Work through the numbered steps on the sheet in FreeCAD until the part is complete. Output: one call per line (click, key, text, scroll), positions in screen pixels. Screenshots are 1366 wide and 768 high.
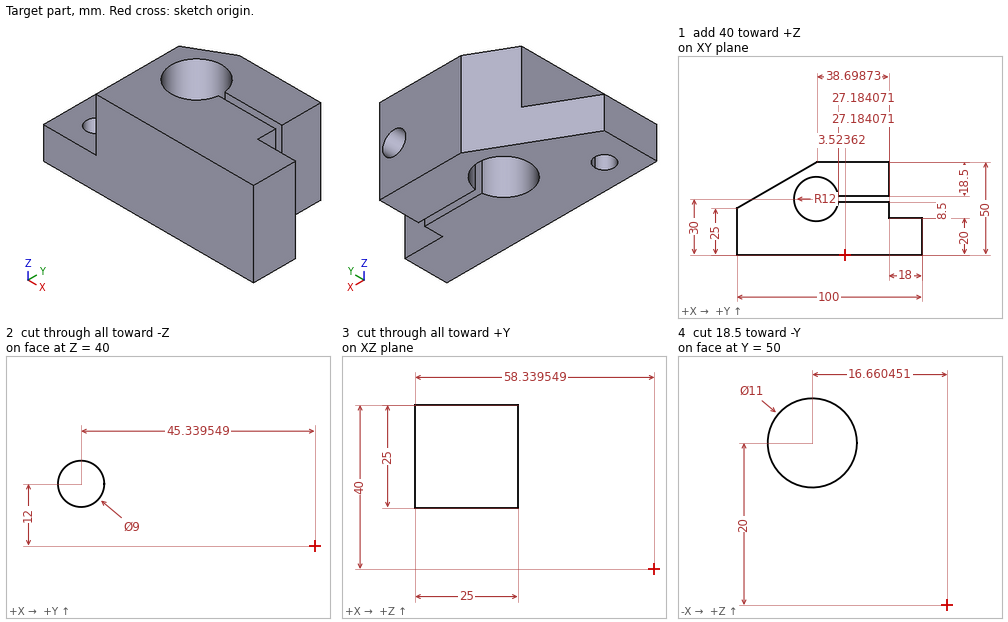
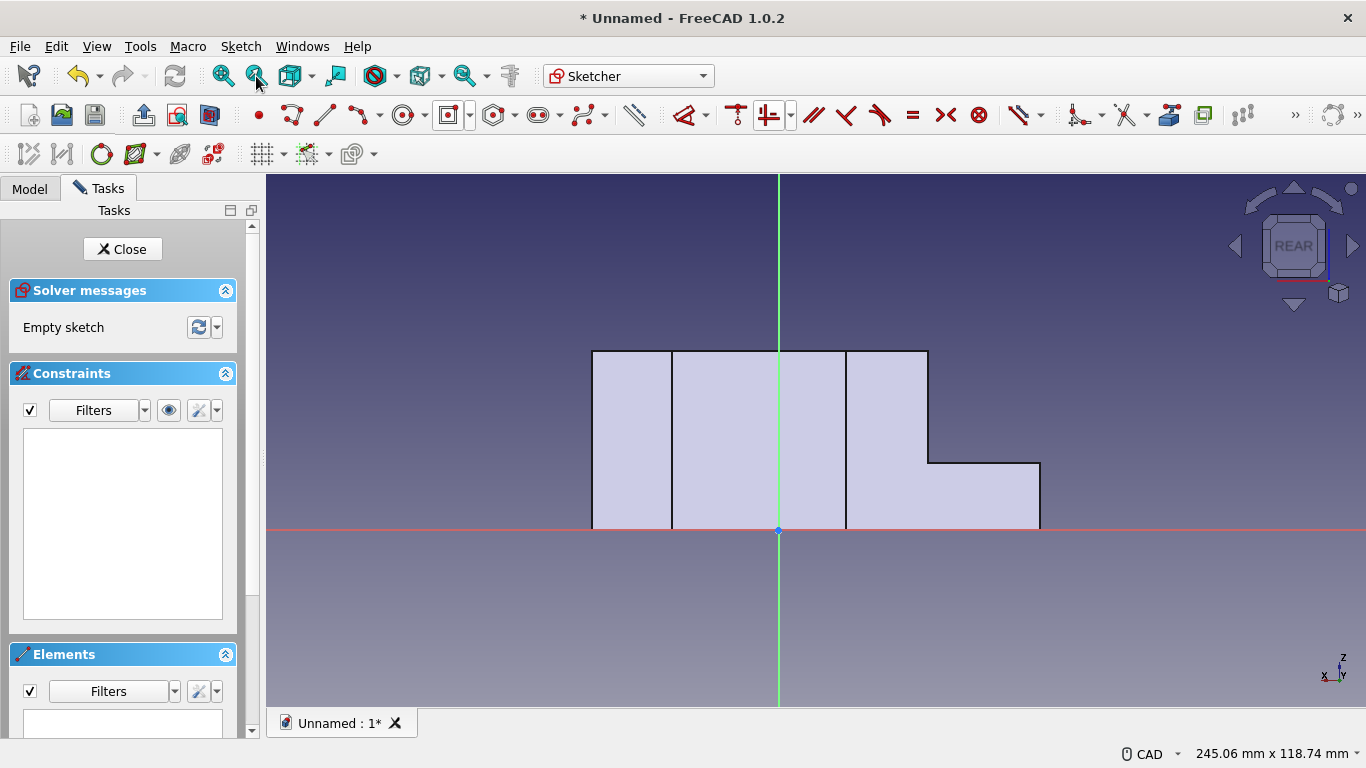
scroll(718, 492, up, 5)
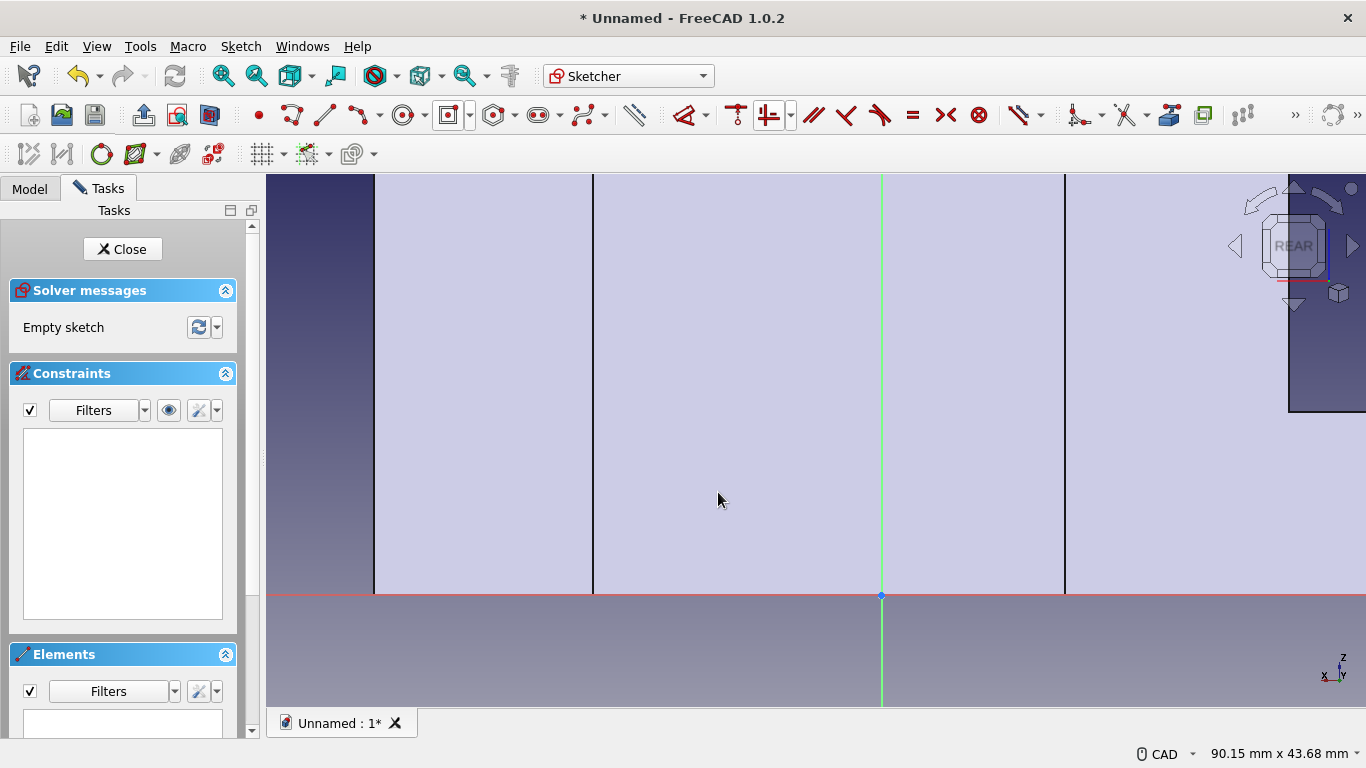
key(g)
key(c)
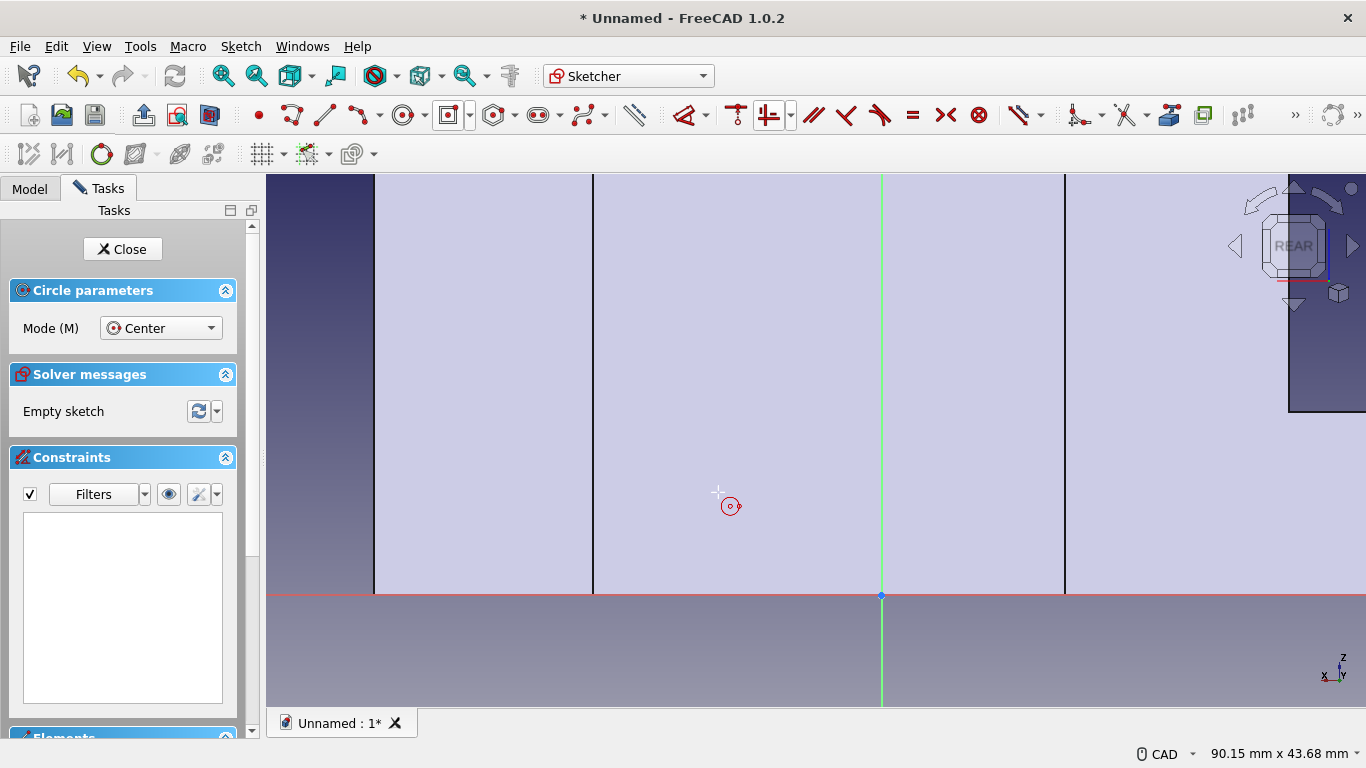
click(679, 351)
move(726, 304)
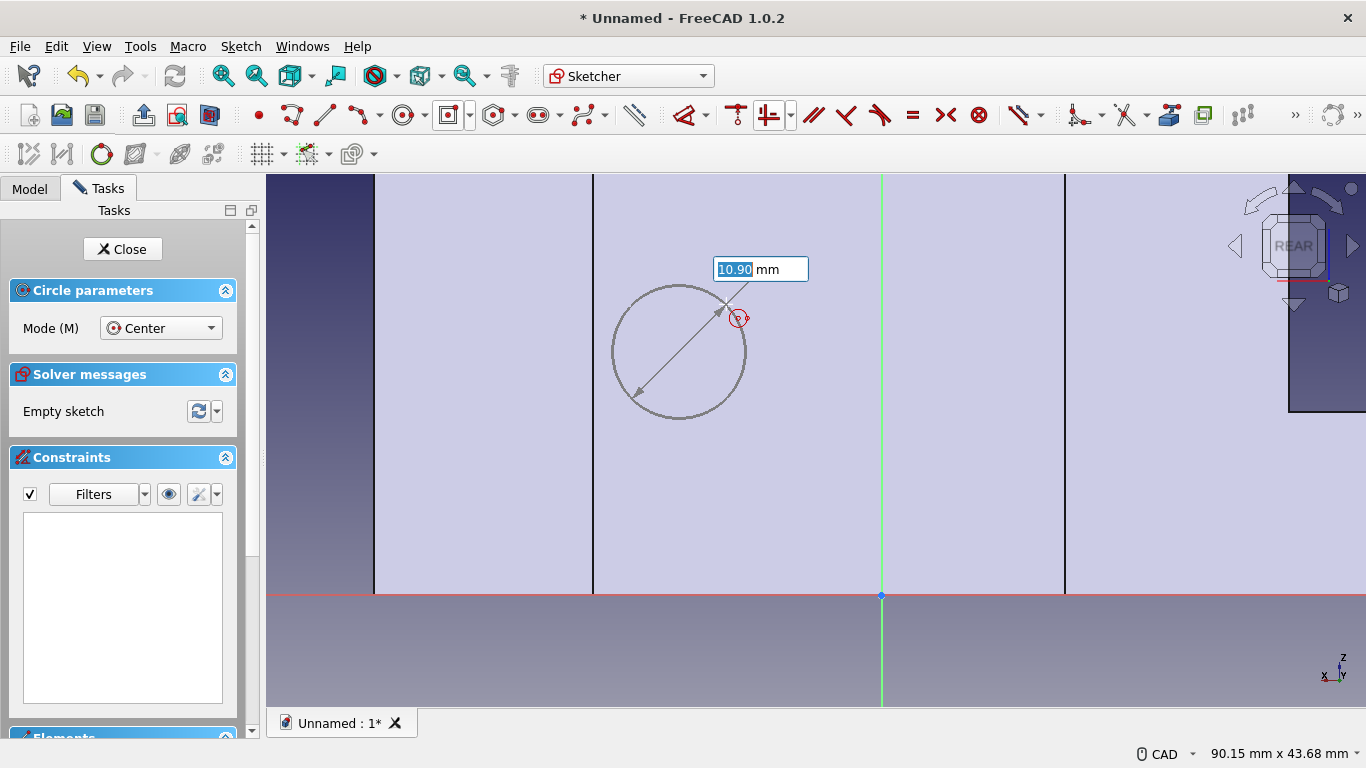
text(11)
key(Return)
key(Escape)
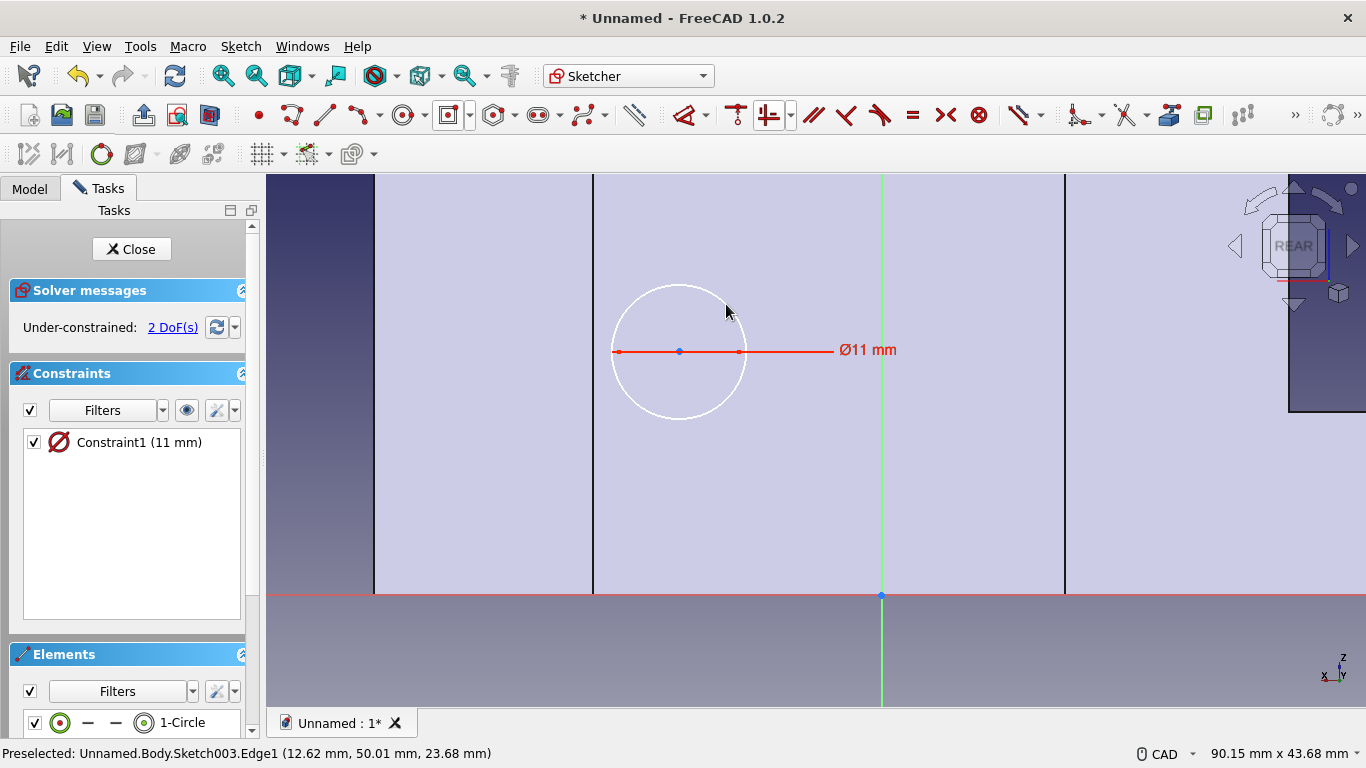
click(684, 116)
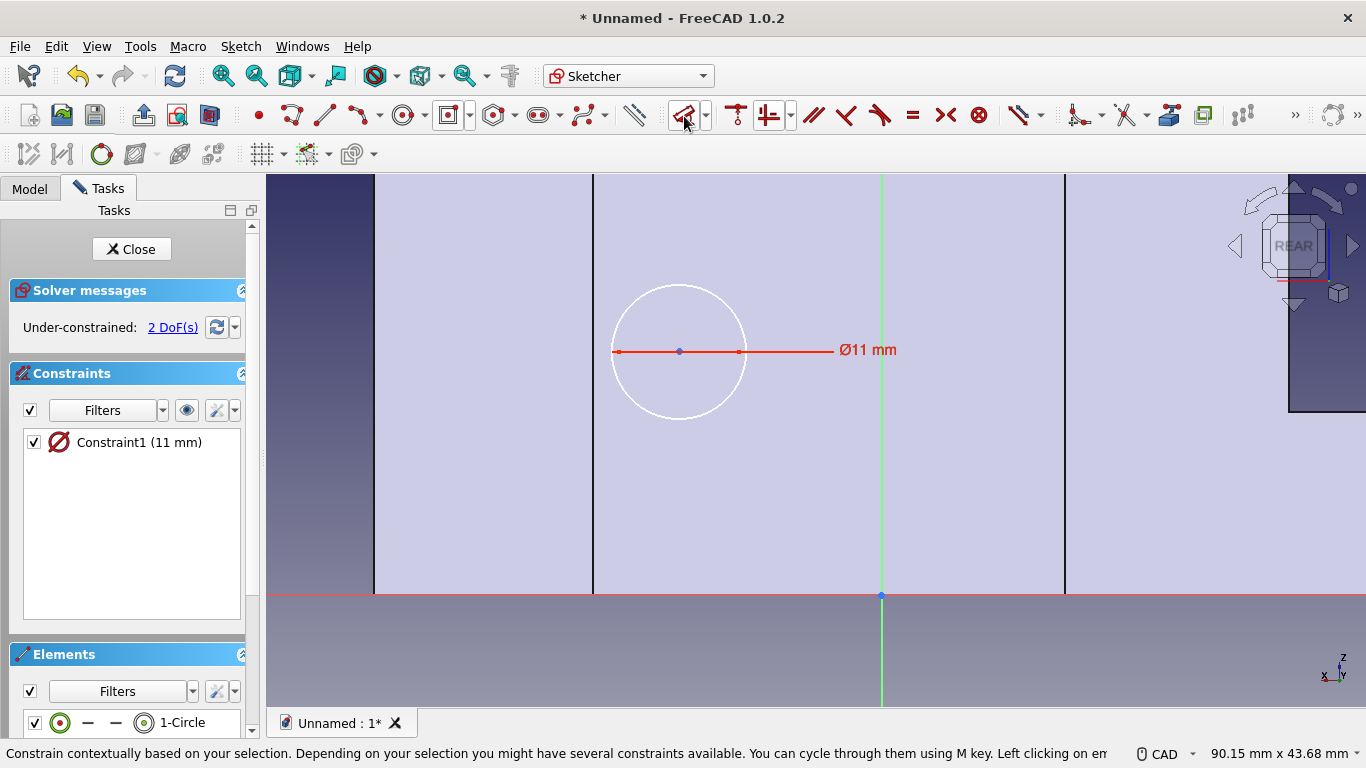
click(679, 352)
click(916, 474)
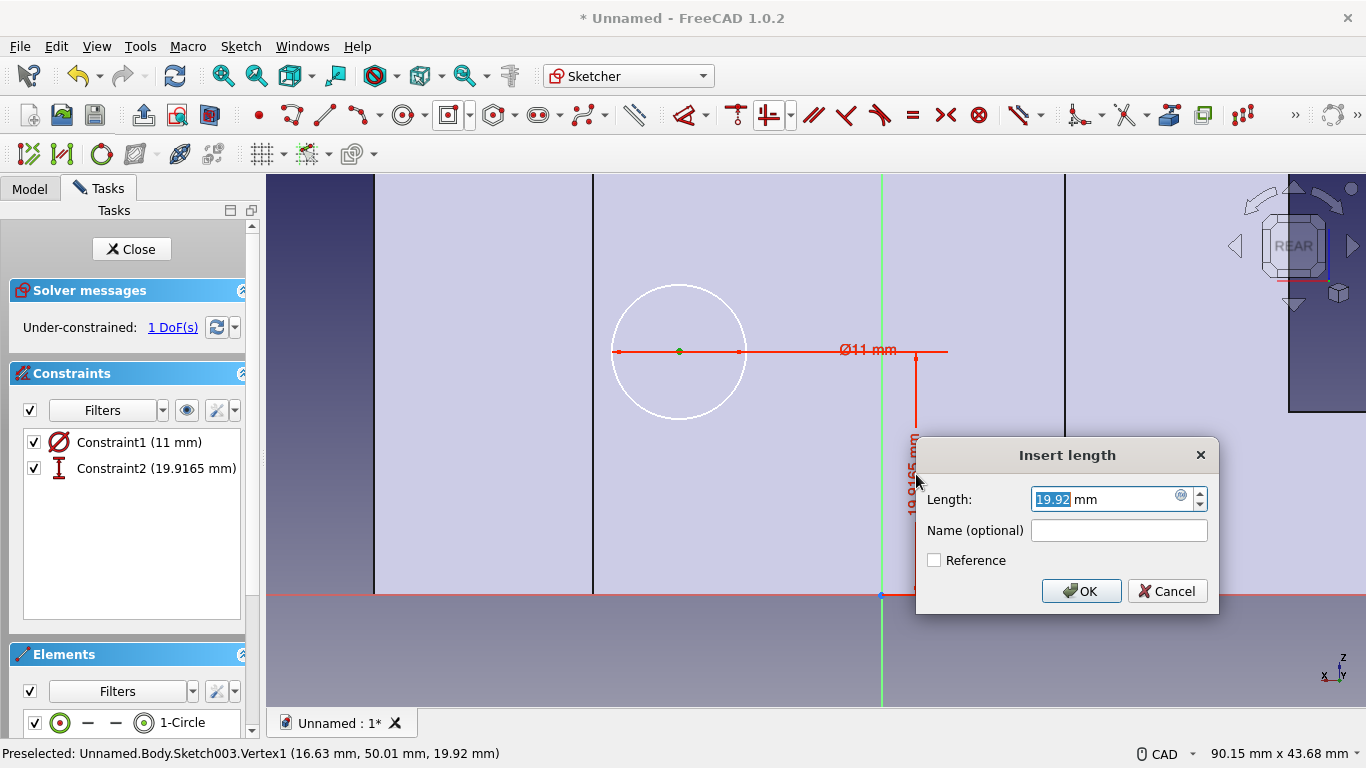
text(20)
key(Return)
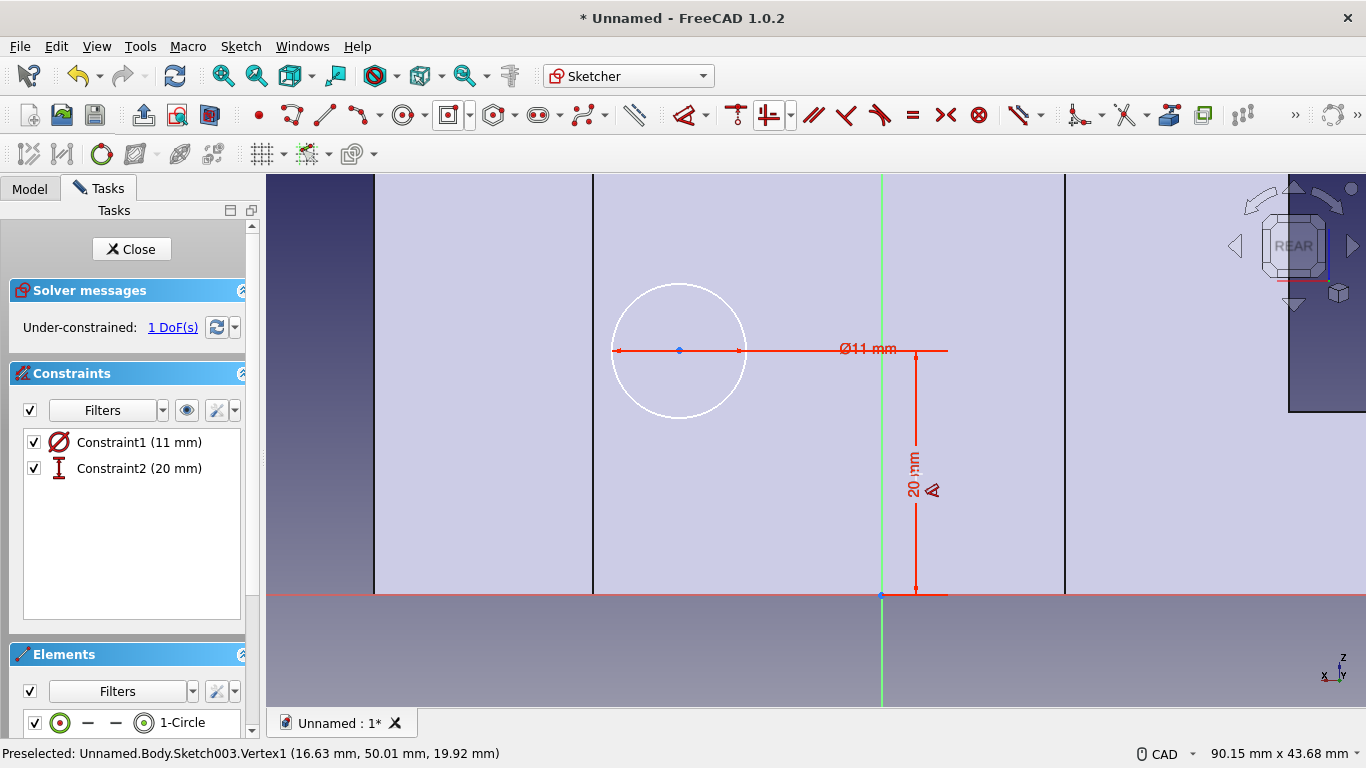
click(679, 351)
click(780, 629)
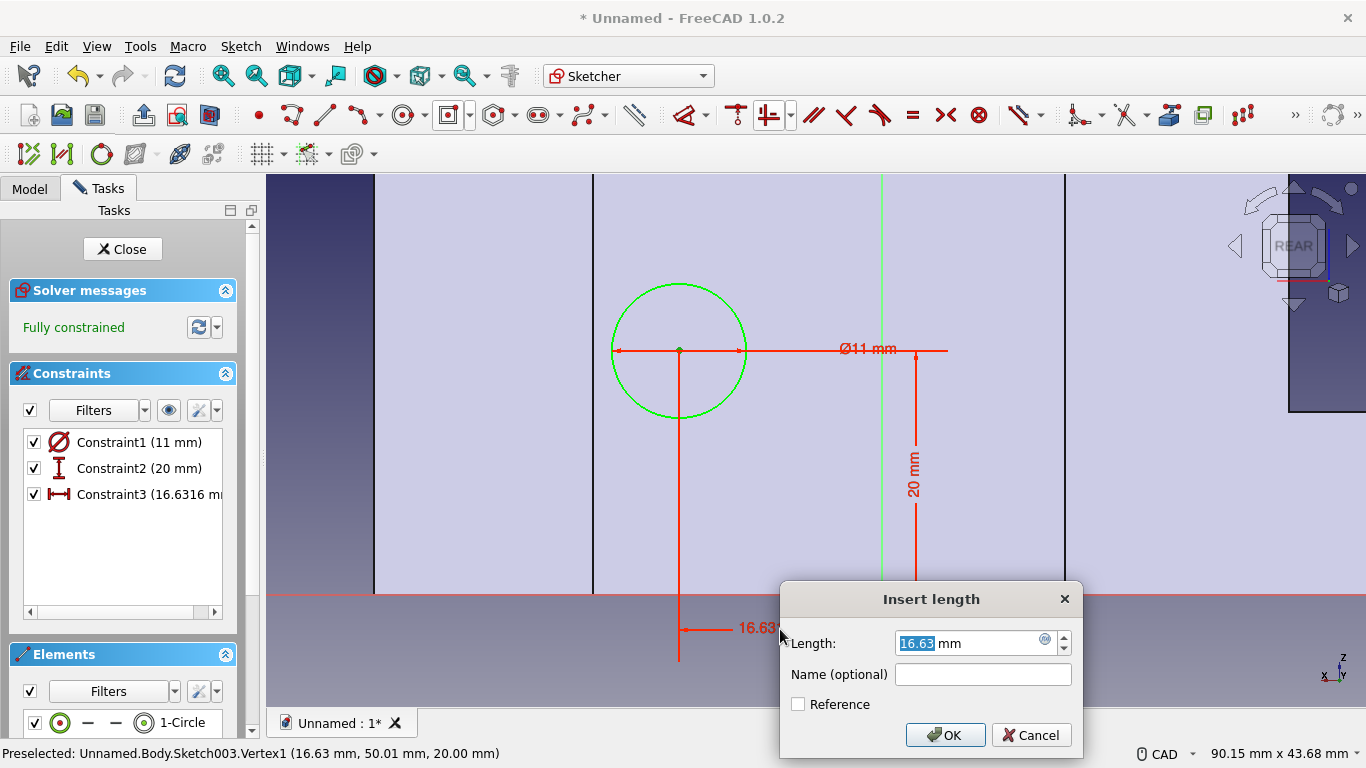
text(16.660451)
key(Return)
key(Escape)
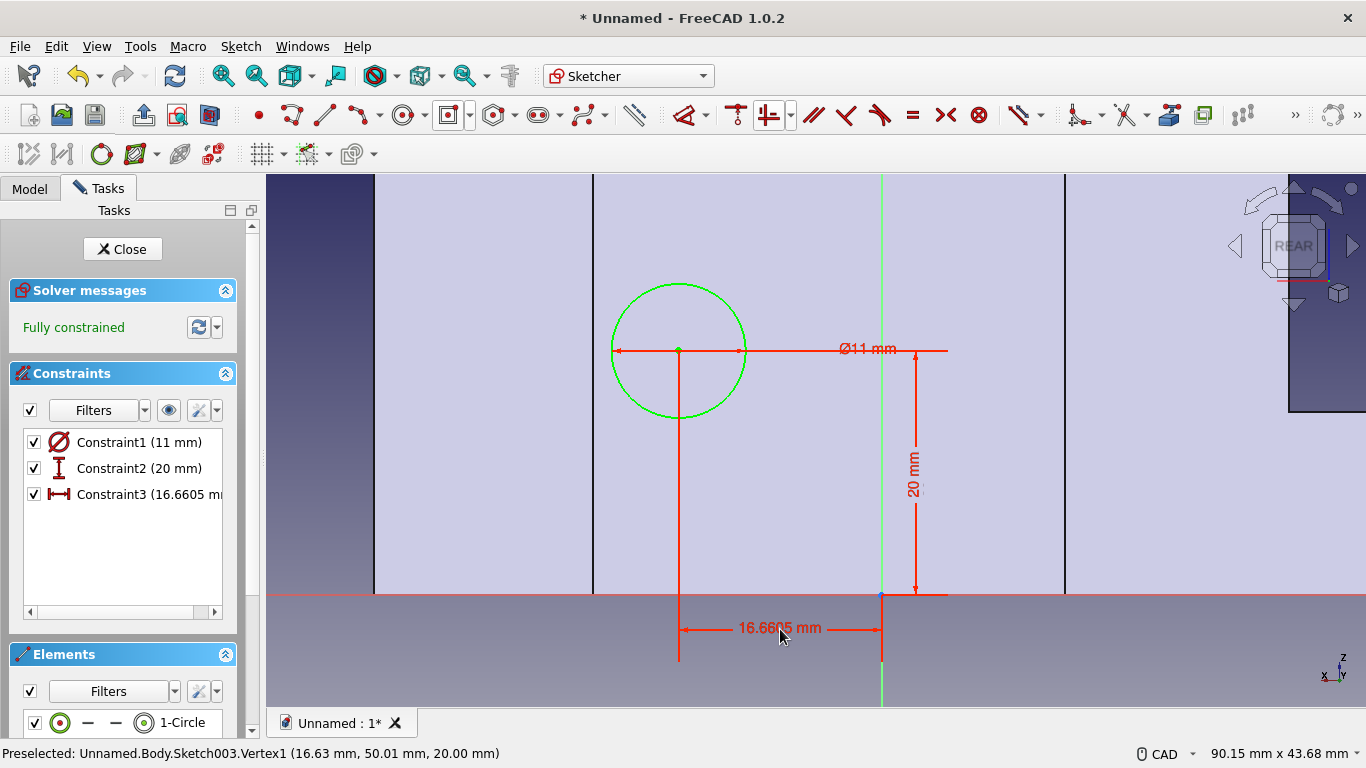
click(123, 249)